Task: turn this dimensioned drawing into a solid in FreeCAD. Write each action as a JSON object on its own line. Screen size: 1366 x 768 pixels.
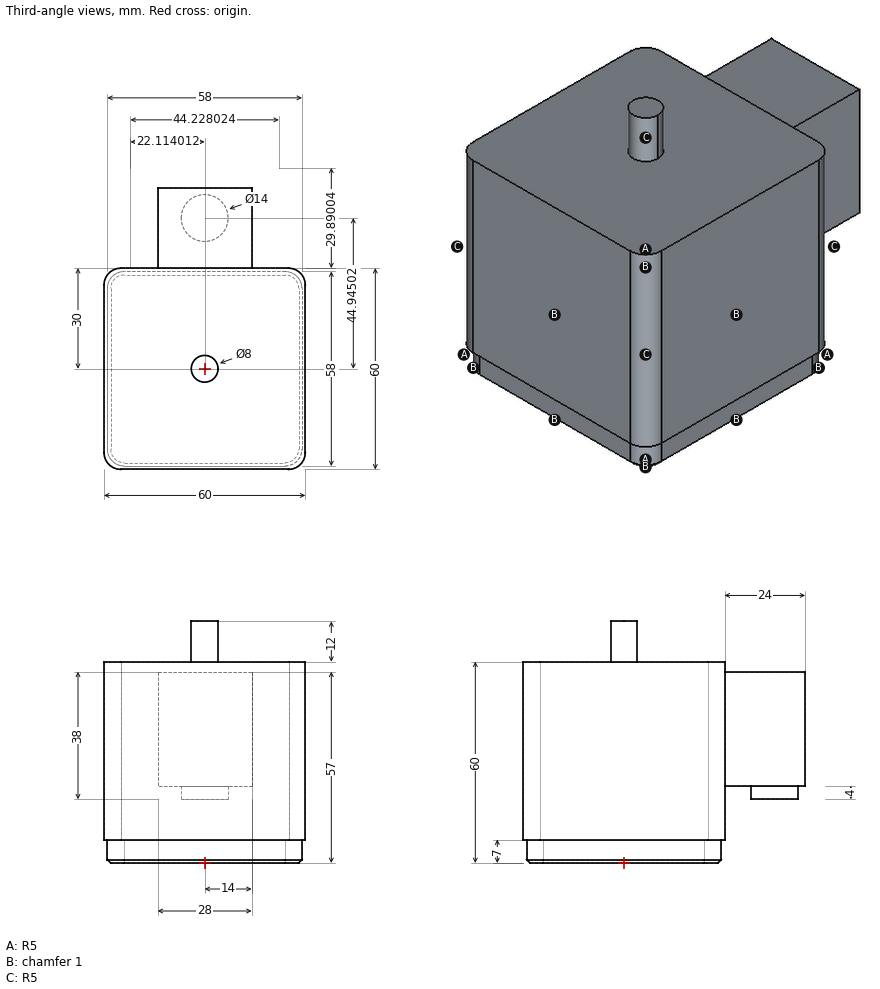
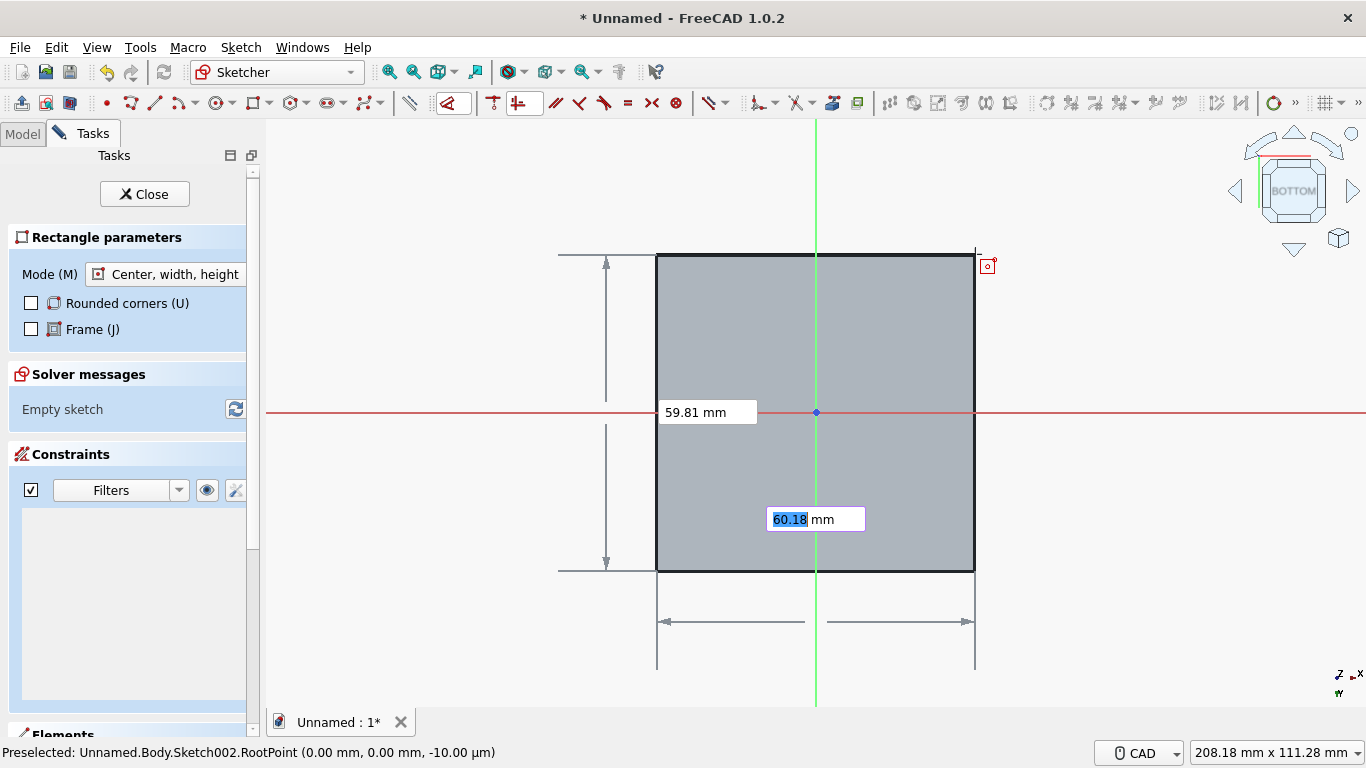
{"action": "type", "text": "60"}
{"action": "key", "text": "Tab"}
{"action": "type", "text": "60"}
{"action": "key", "text": "Return"}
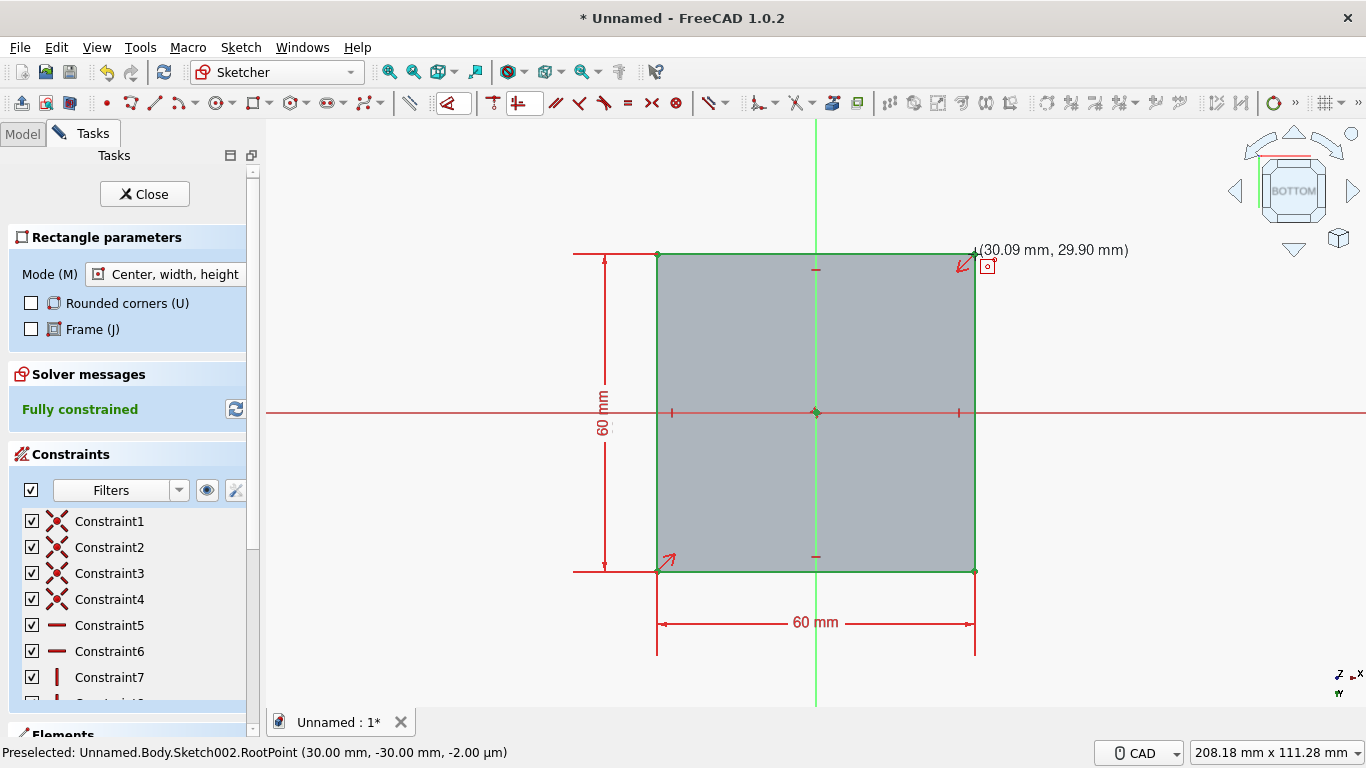
{"action": "left_click", "coordinate": [816, 413]}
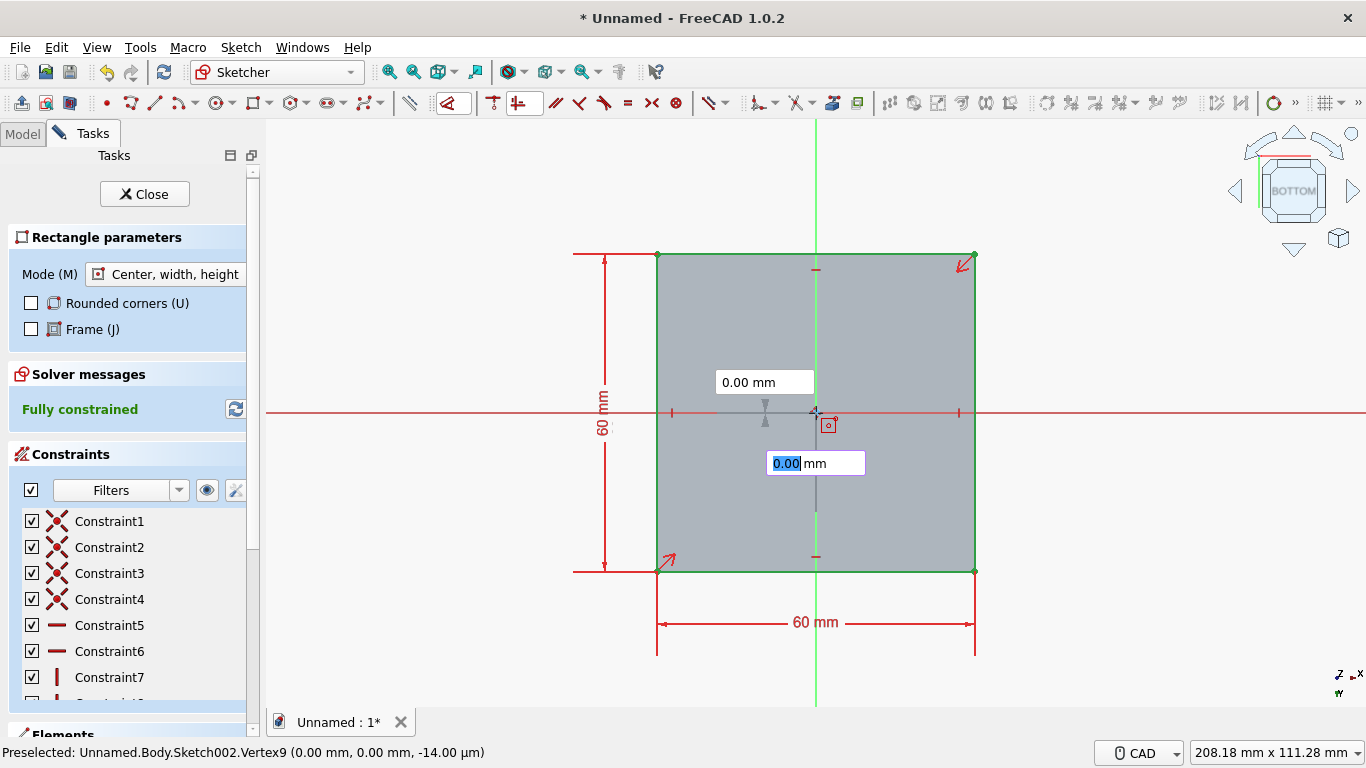
{"action": "scroll", "coordinate": [969, 260], "scroll_direction": "up", "scroll_amount": 6}
{"action": "mouse_move", "coordinate": [968, 259]}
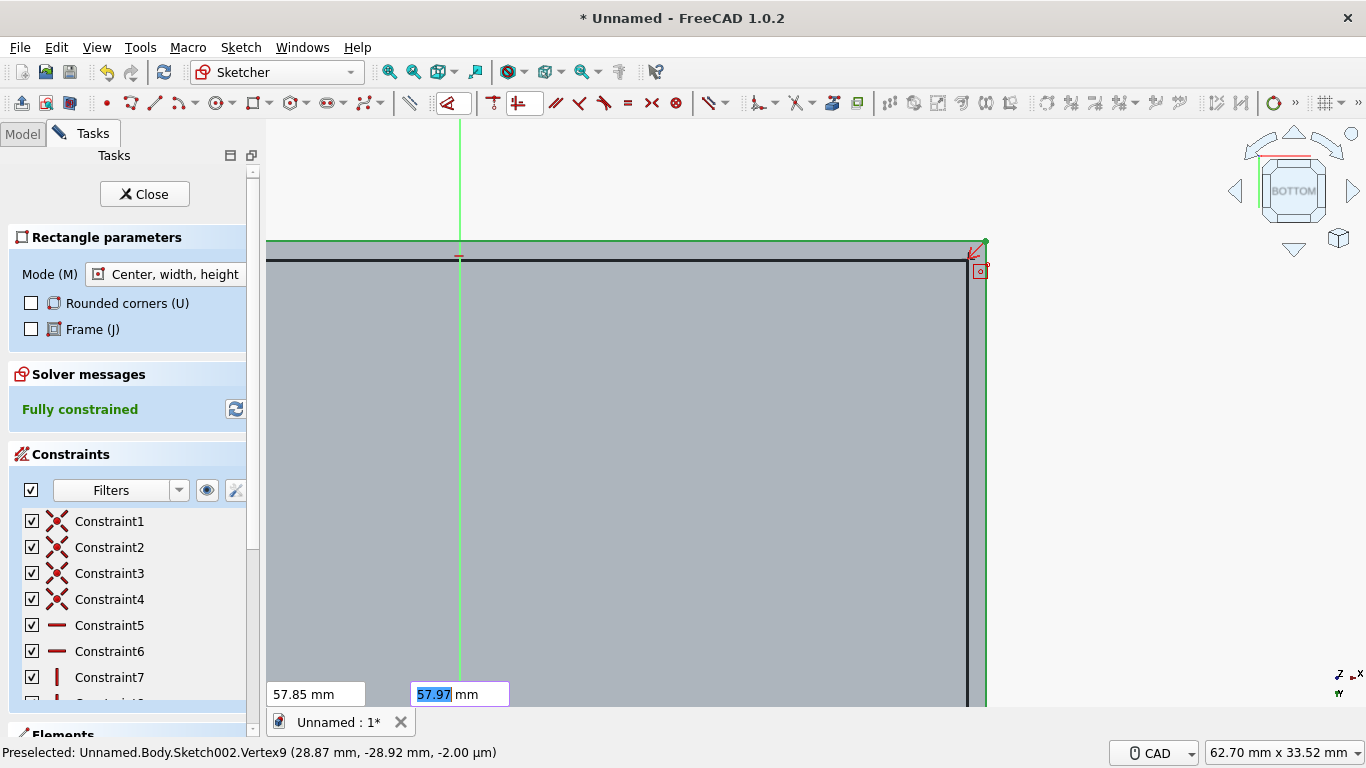
{"action": "type", "text": "58"}
{"action": "key", "text": "Tab"}
{"action": "type", "text": "58"}
{"action": "key", "text": "Return"}
{"action": "key", "text": "Escape"}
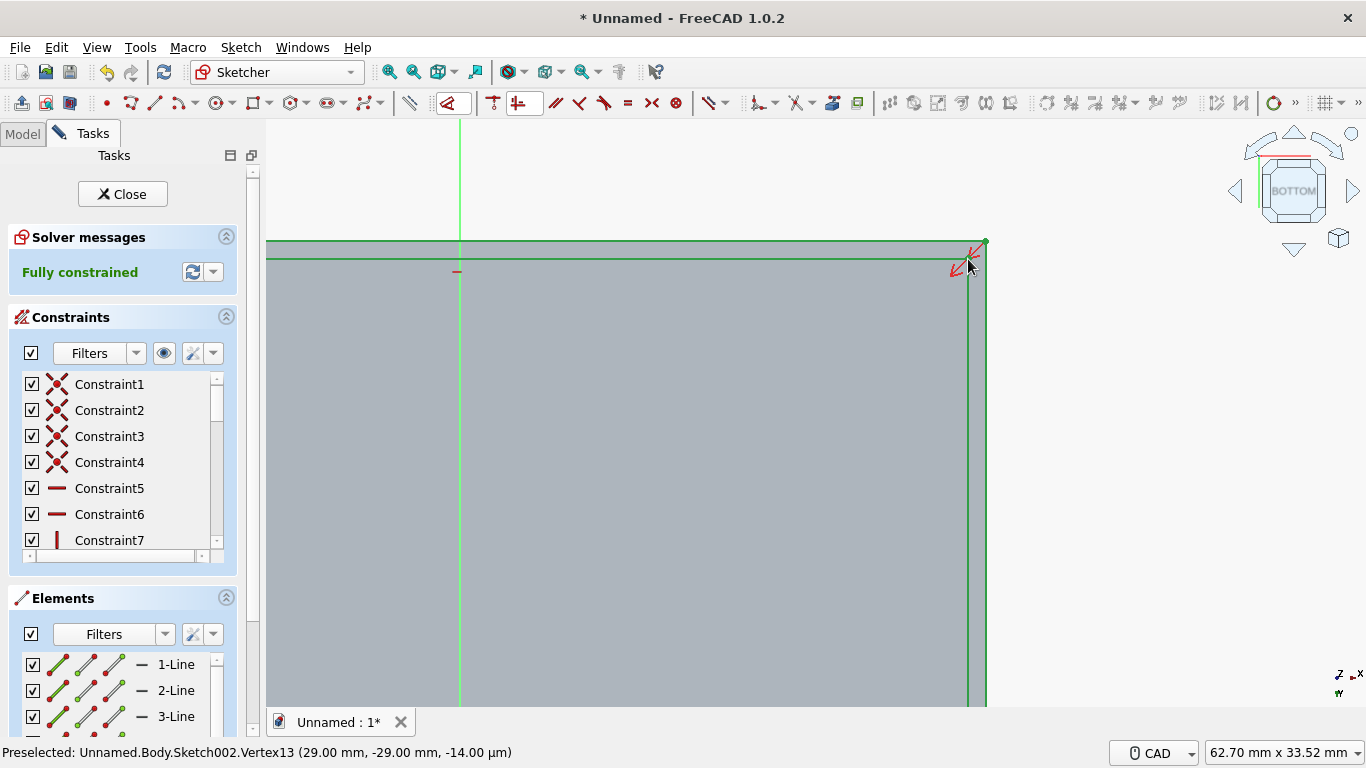
{"action": "left_click", "coordinate": [123, 194]}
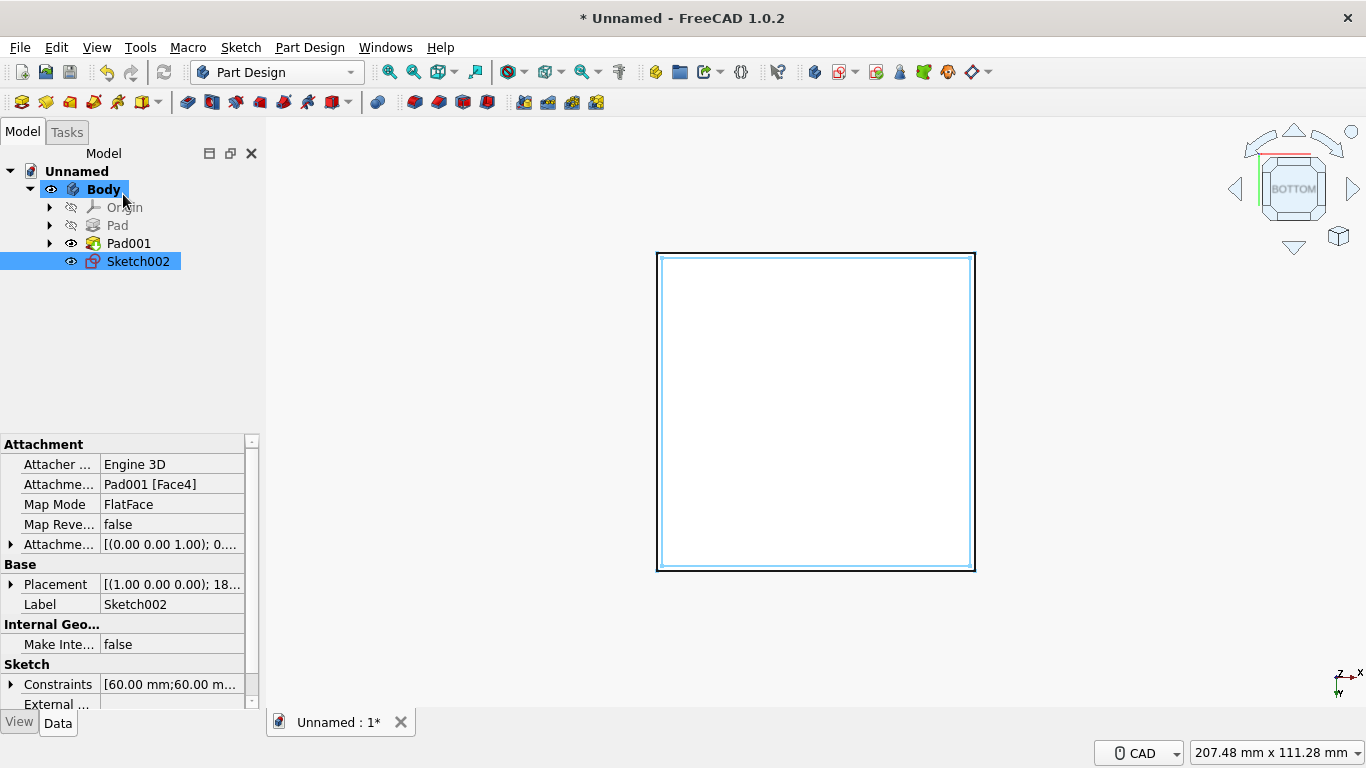
{"action": "left_click", "coordinate": [188, 102]}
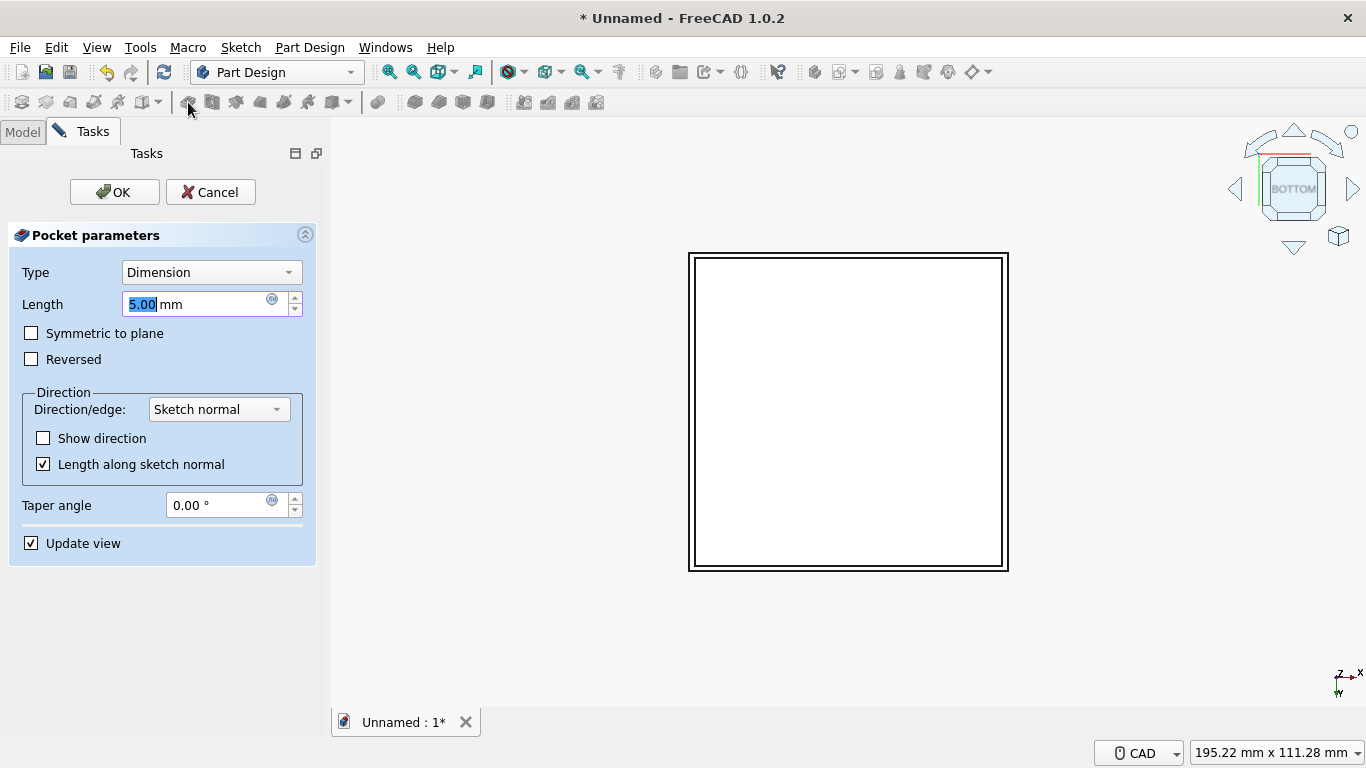
{"action": "type", "text": "7"}
{"action": "key", "text": "Tab"}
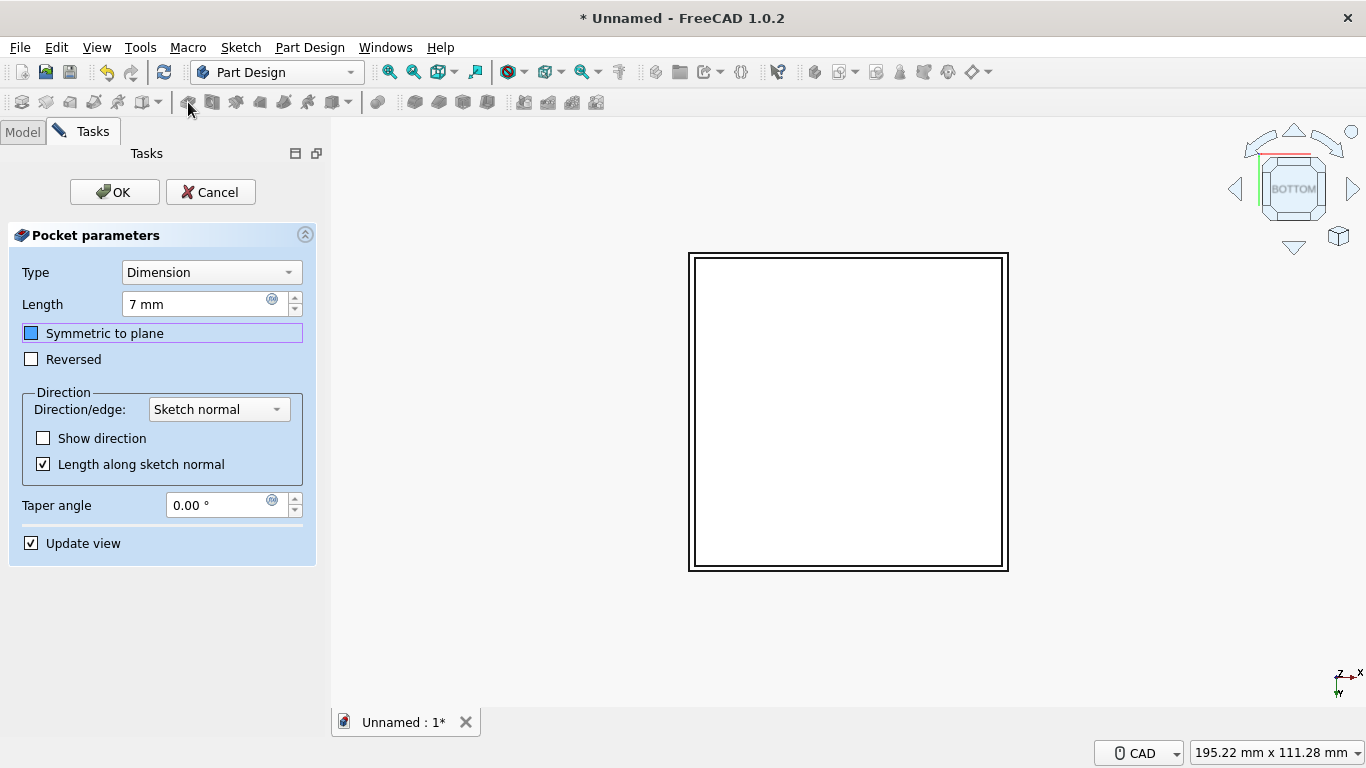
{"action": "left_click", "coordinate": [115, 192]}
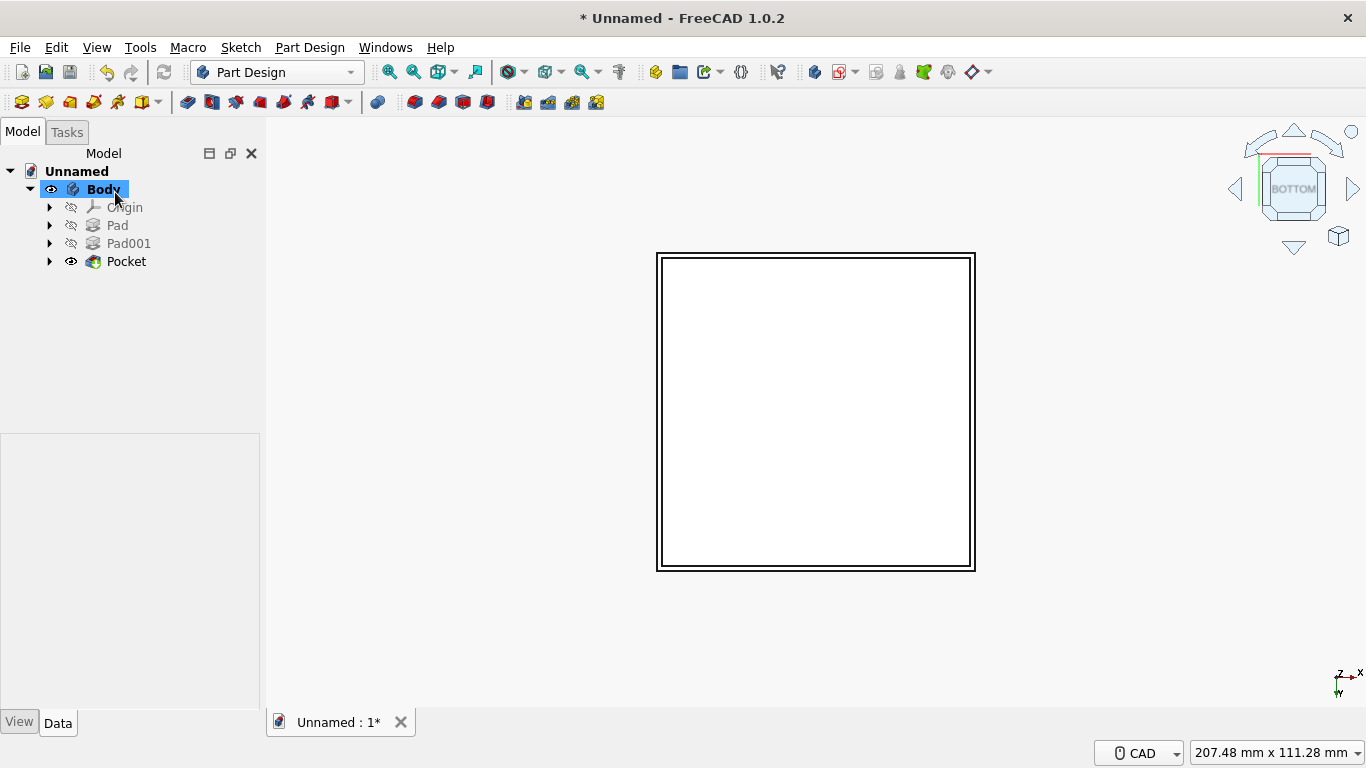
{"action": "key", "text": "0"}